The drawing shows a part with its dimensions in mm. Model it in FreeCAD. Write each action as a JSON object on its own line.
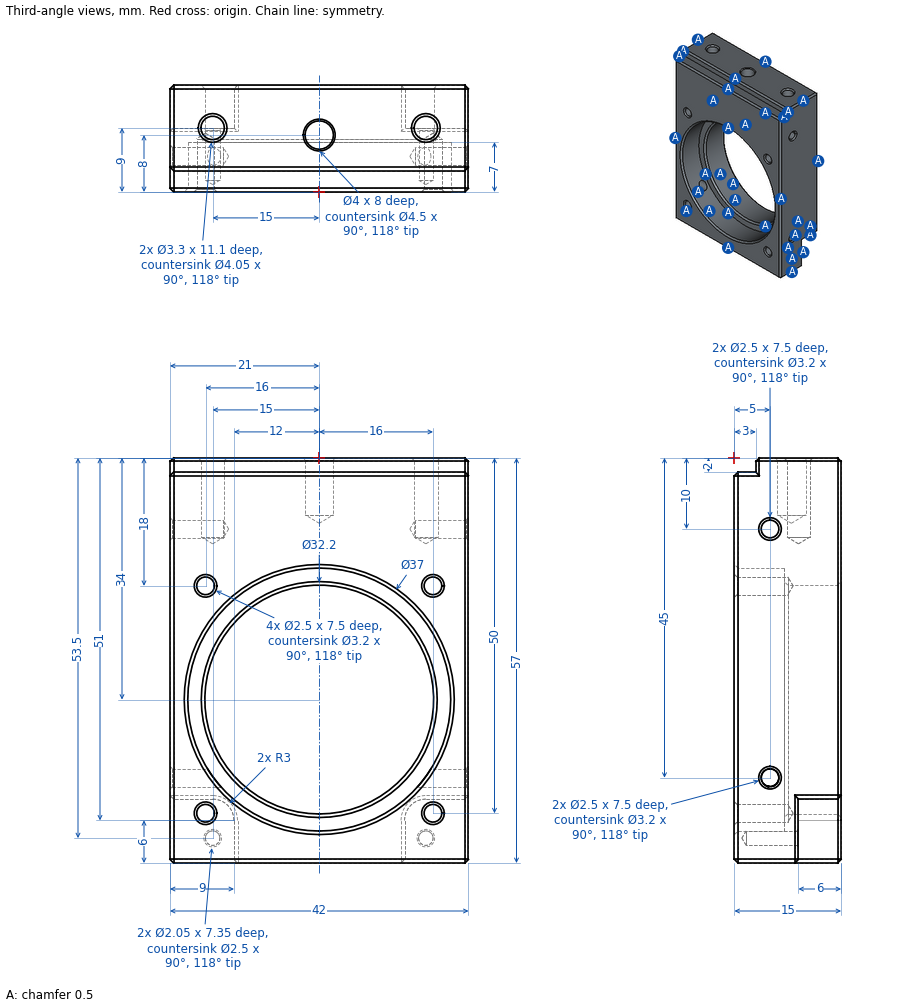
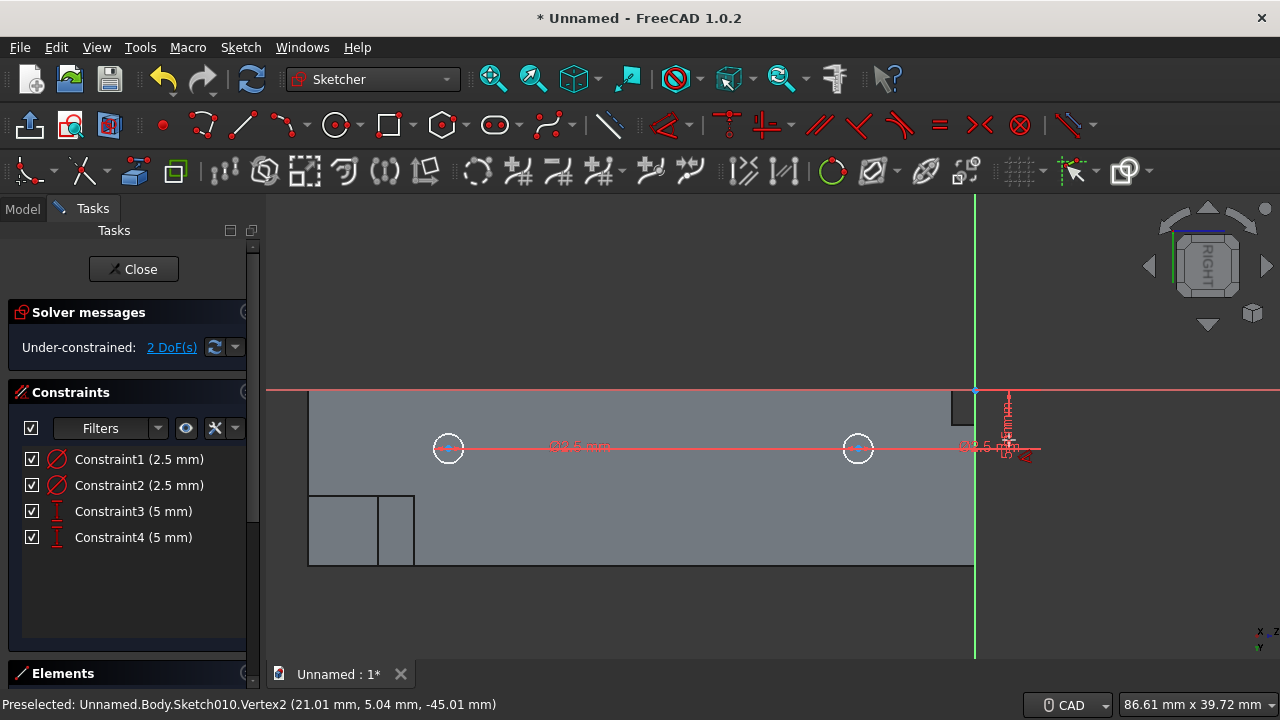
{"action": "left_click", "coordinate": [858, 449]}
{"action": "left_click", "coordinate": [917, 356]}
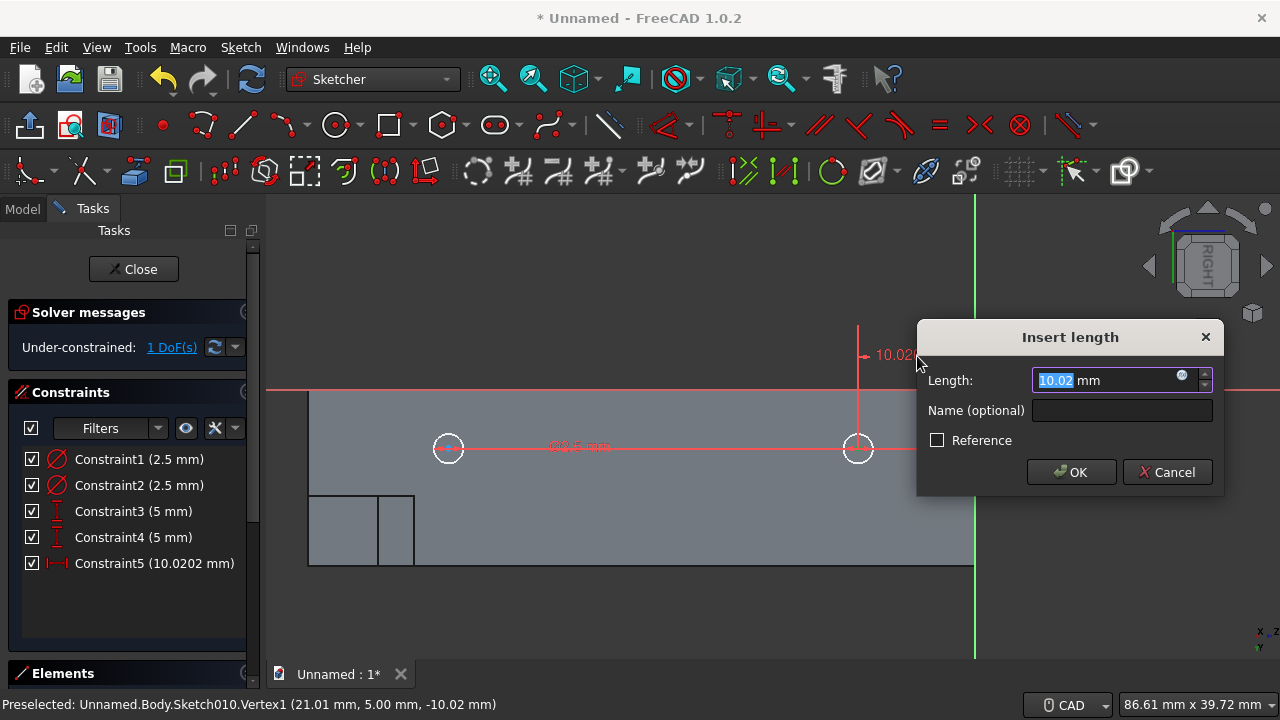
{"action": "type", "text": "10"}
{"action": "key", "text": "Return"}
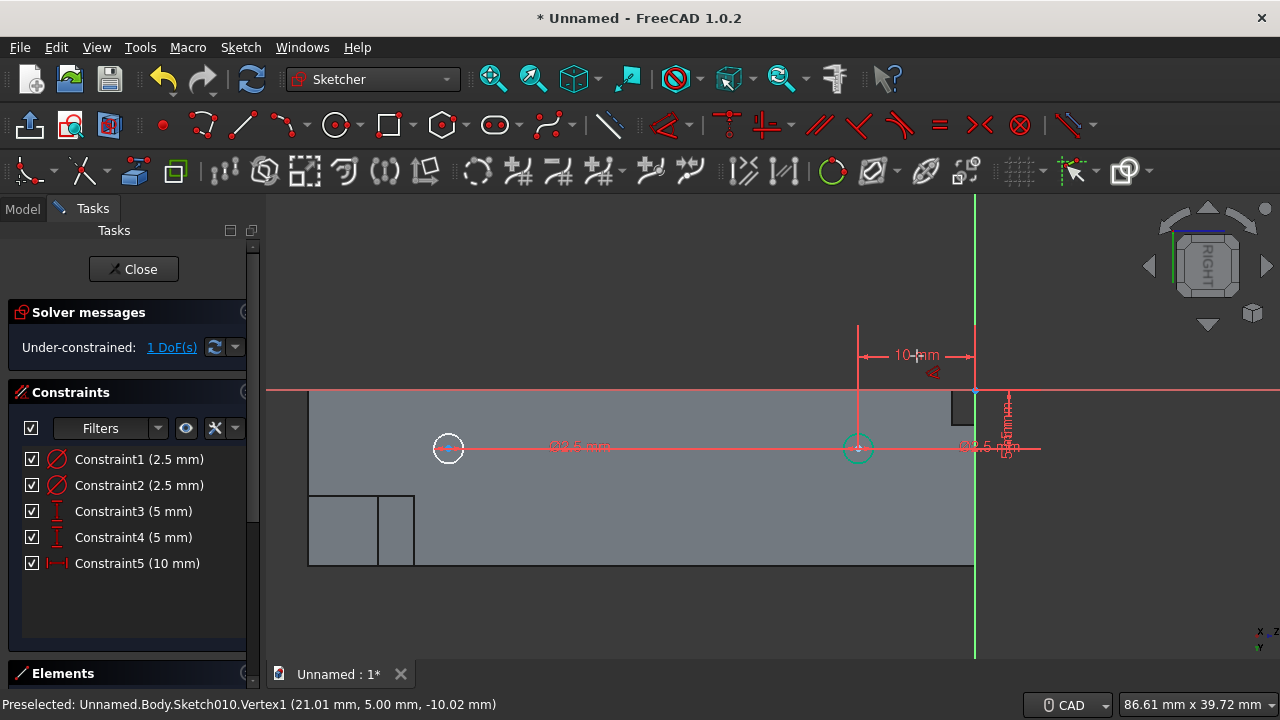
{"action": "left_click", "coordinate": [449, 449]}
{"action": "left_click", "coordinate": [712, 356]}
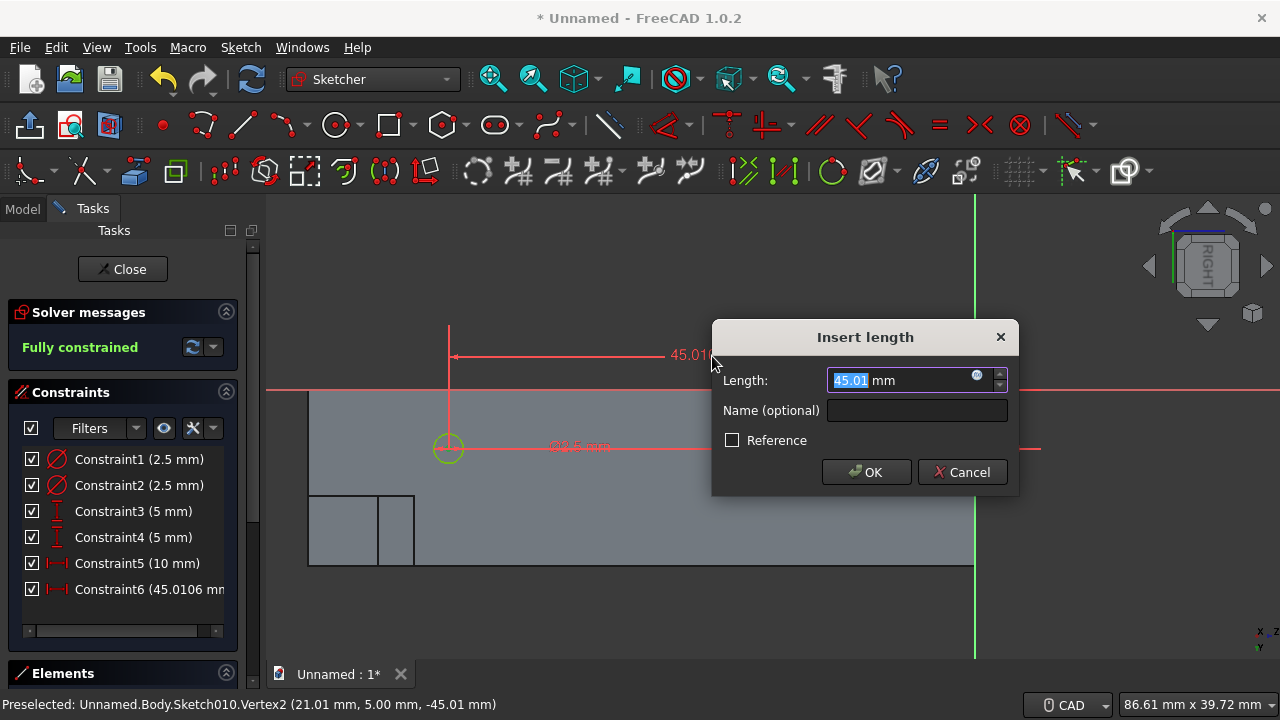
{"action": "type", "text": "45"}
{"action": "key", "text": "Return"}
{"action": "key", "text": "Escape"}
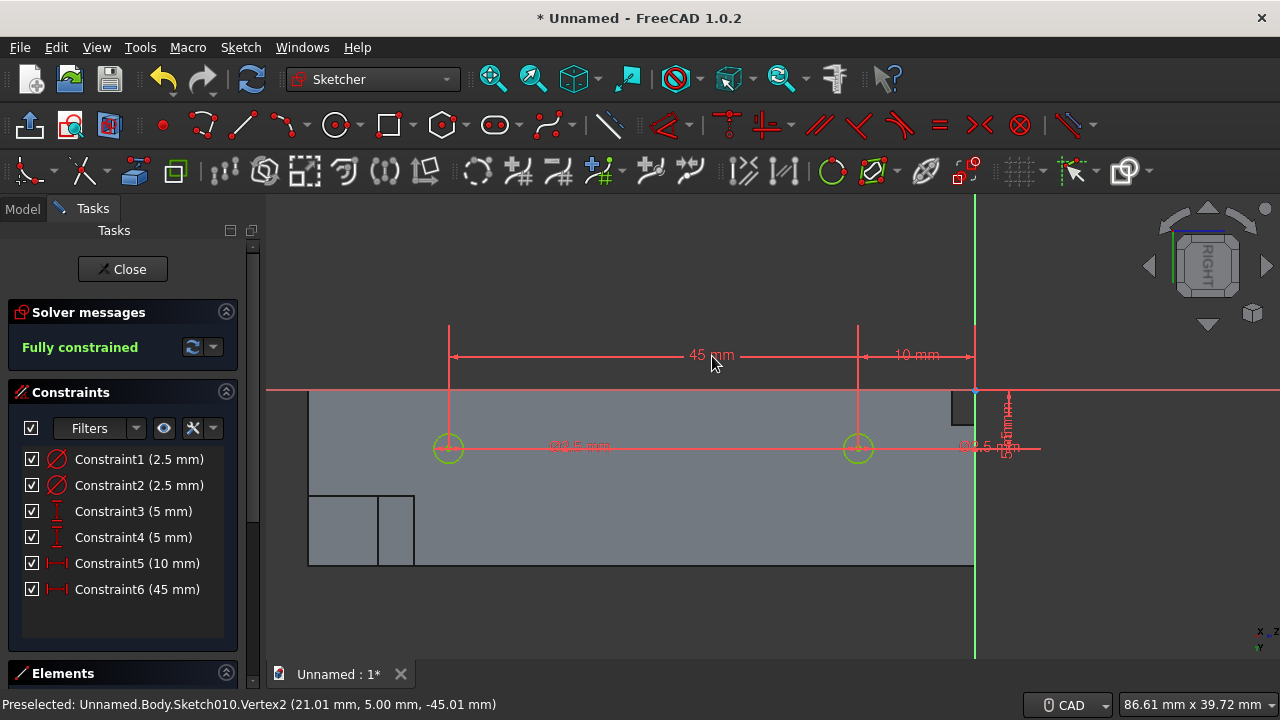
{"action": "left_click", "coordinate": [123, 269]}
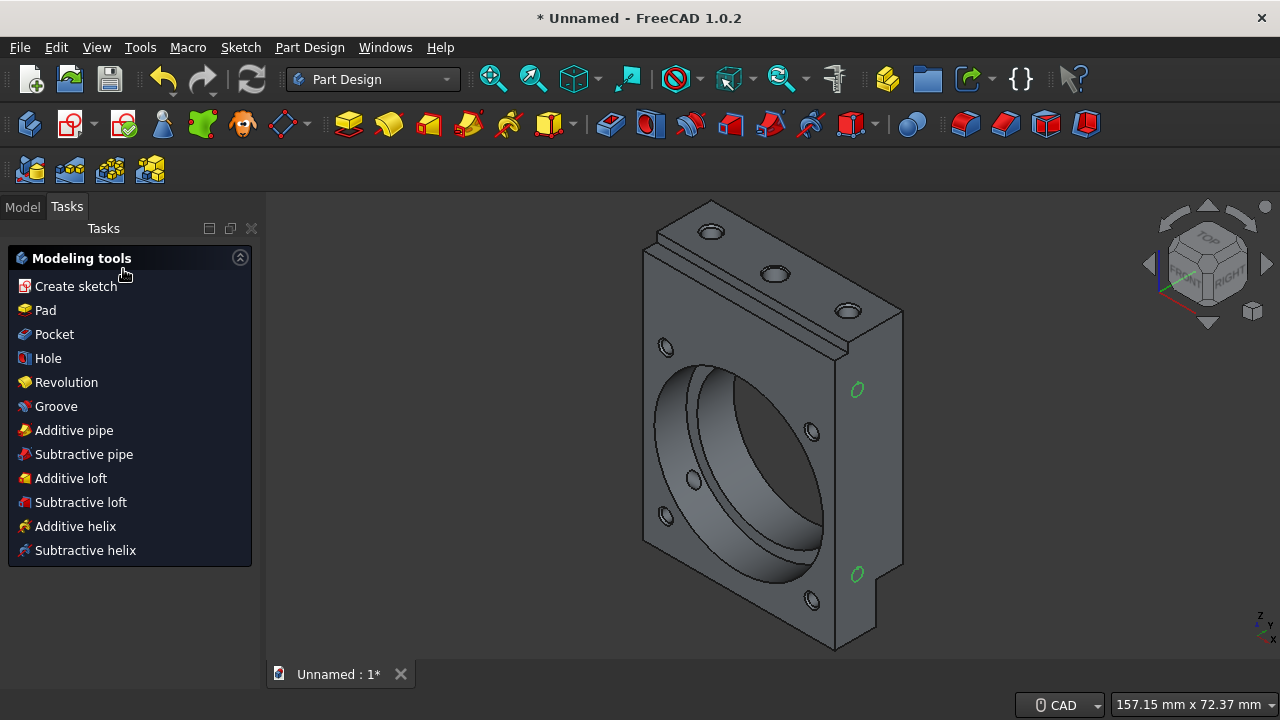
{"action": "left_click", "coordinate": [652, 124]}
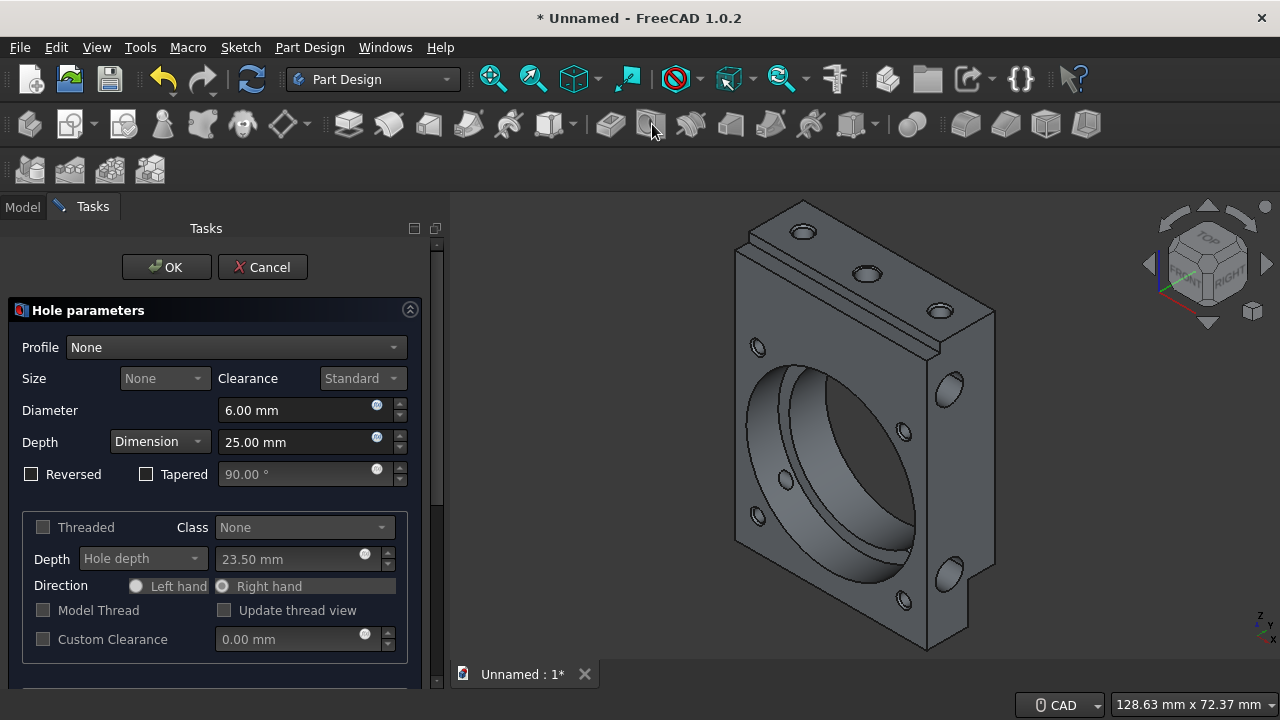
{"action": "triple_click", "coordinate": [305, 410]}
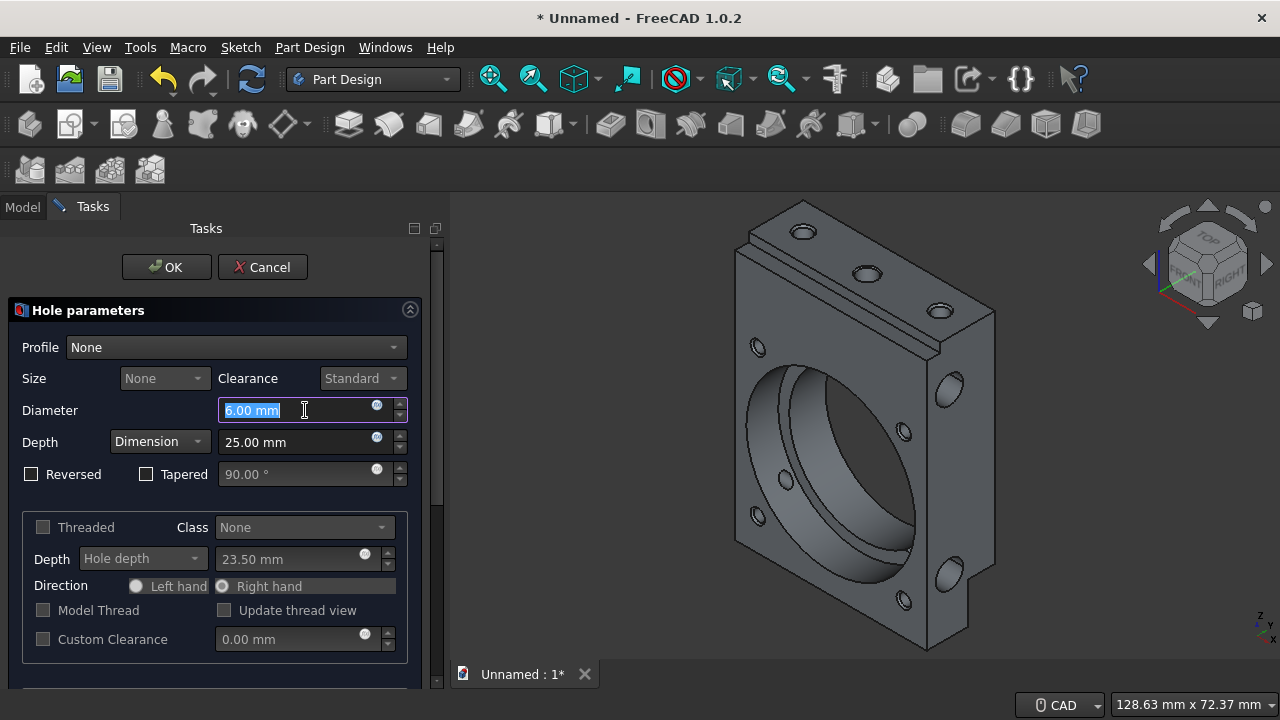
{"action": "type", "text": "2.5"}
{"action": "key", "text": "Tab"}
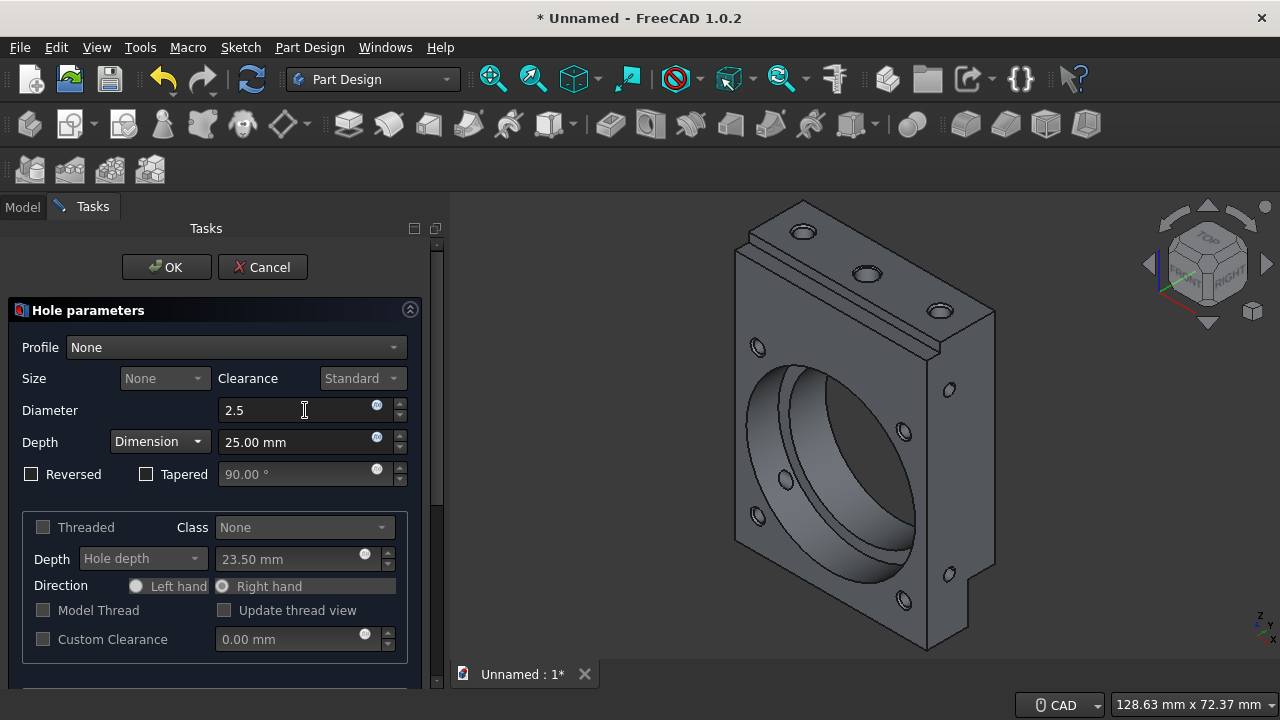
{"action": "triple_click", "coordinate": [305, 442]}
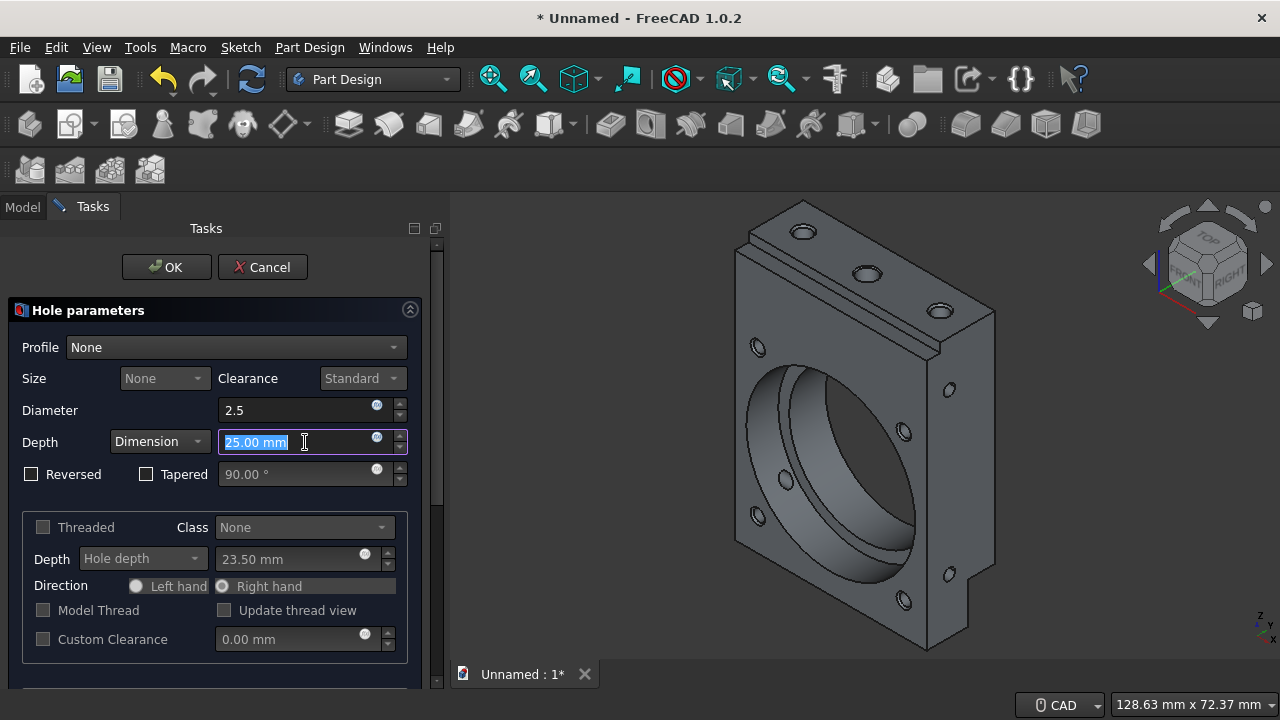
{"action": "type", "text": "7.5"}
{"action": "key", "text": "Tab"}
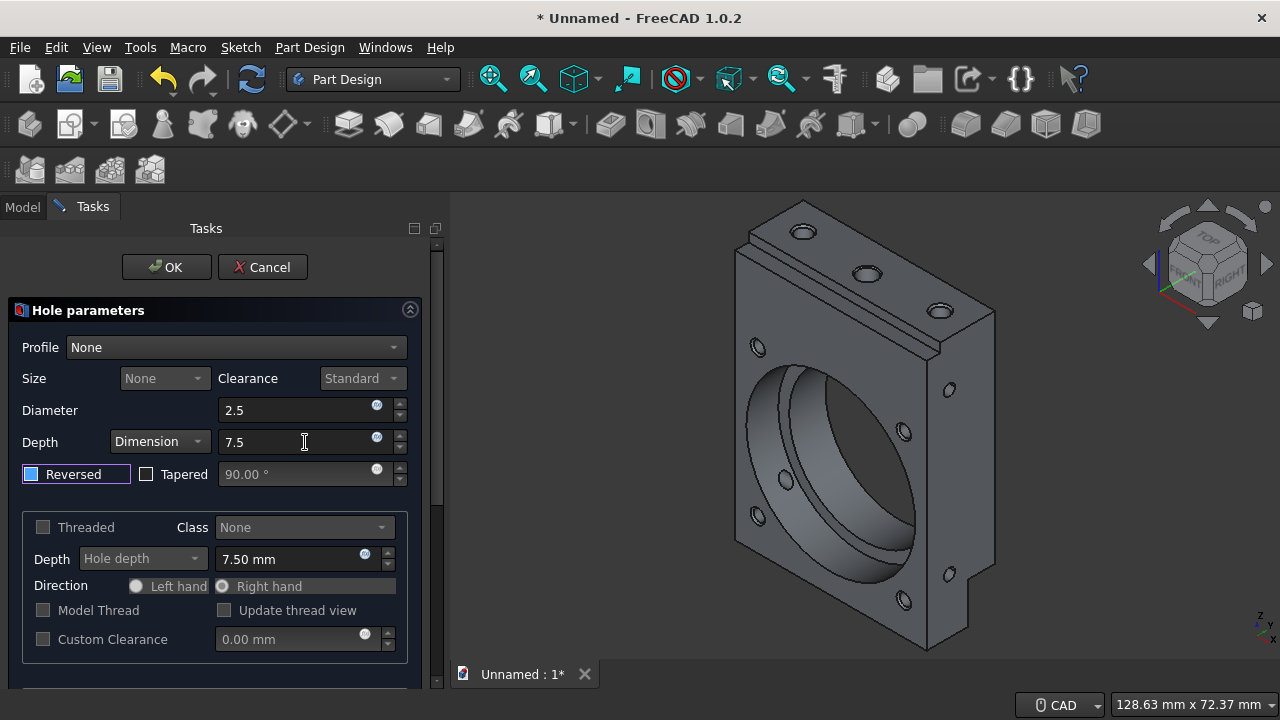
{"action": "scroll", "coordinate": [437, 463], "scroll_direction": "down", "scroll_amount": 2}